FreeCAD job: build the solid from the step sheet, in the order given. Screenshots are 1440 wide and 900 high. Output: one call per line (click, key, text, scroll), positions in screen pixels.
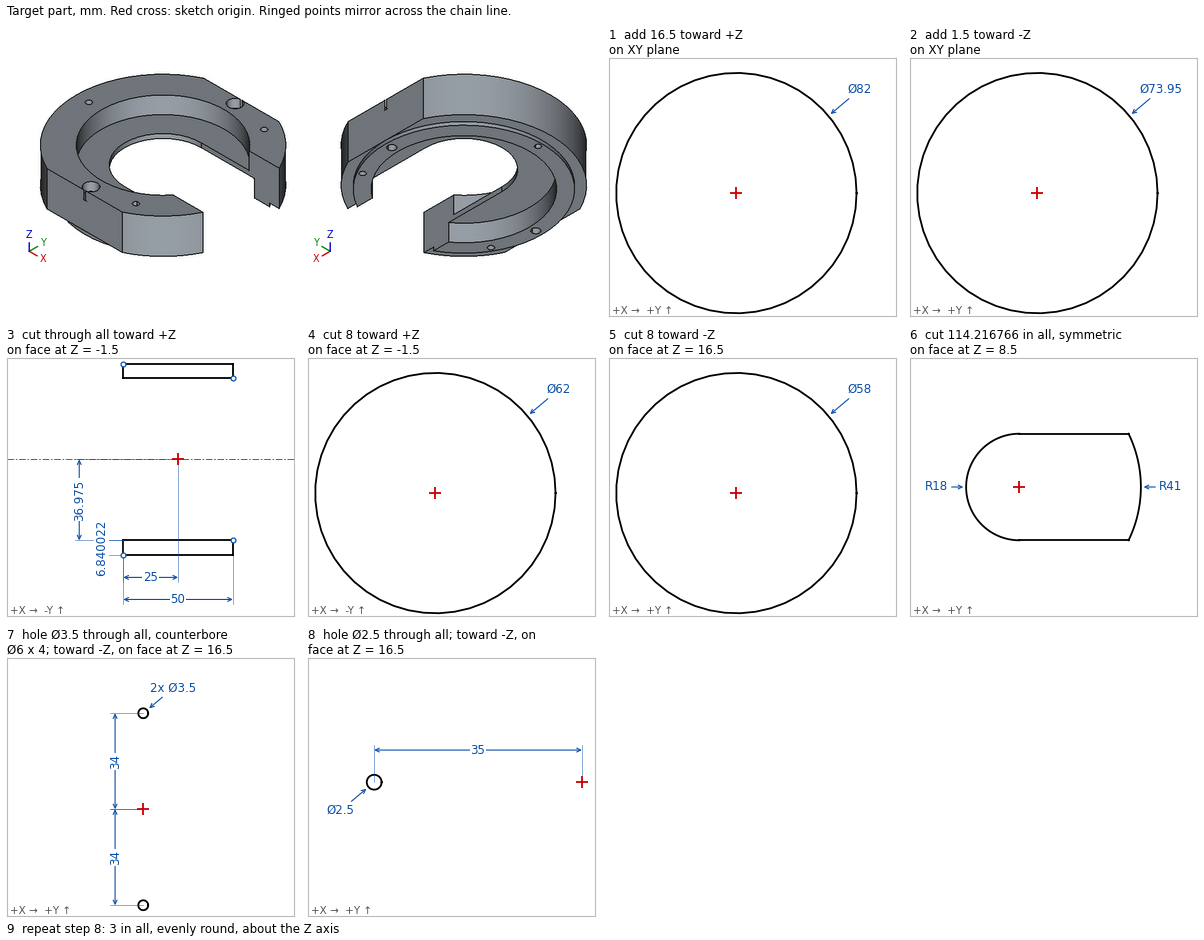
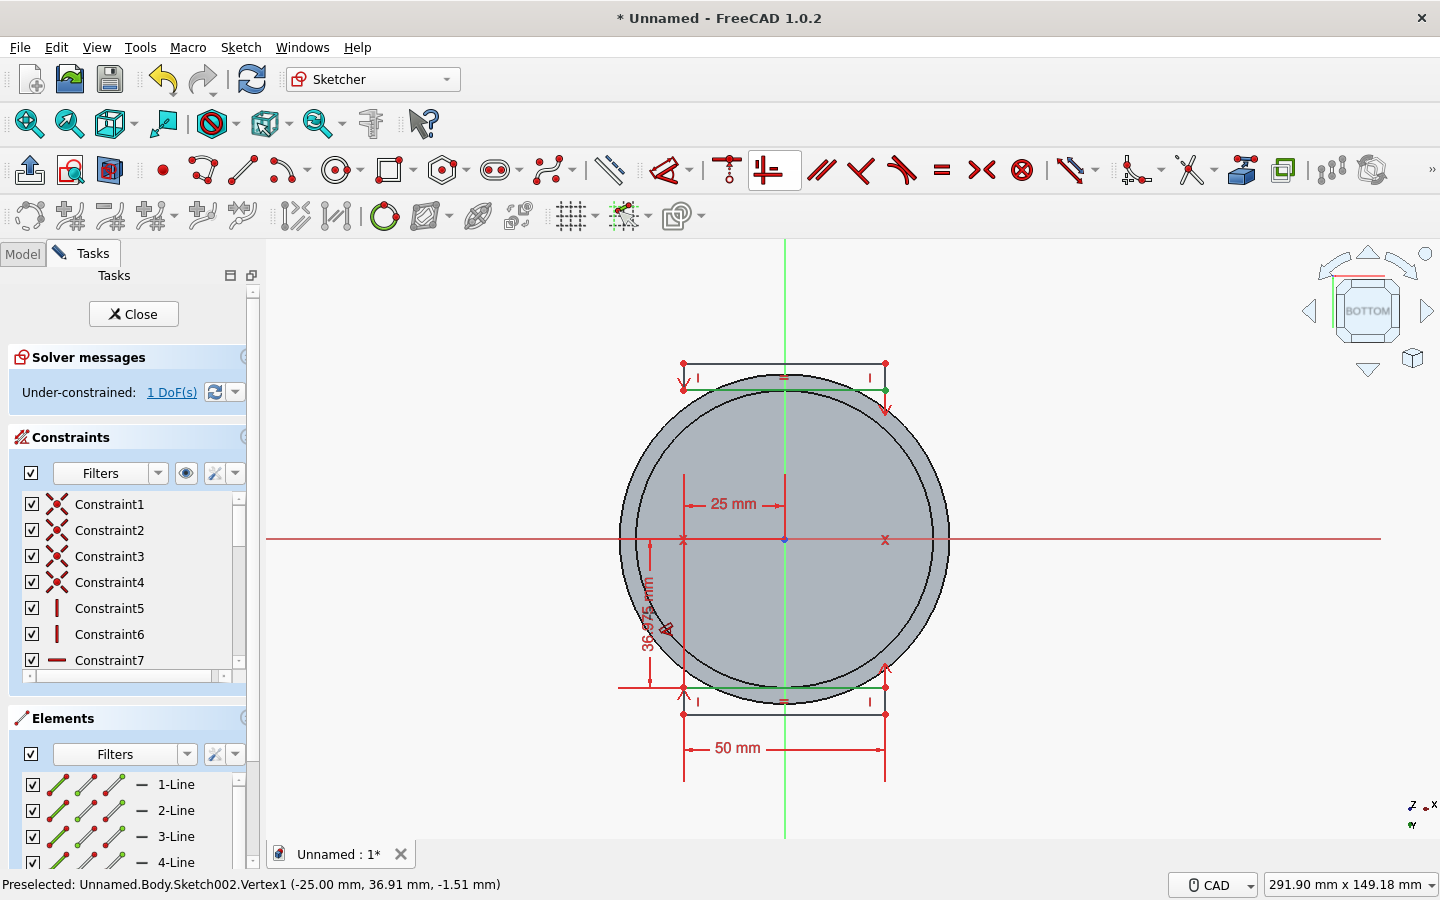
scroll(684, 699, up, 2)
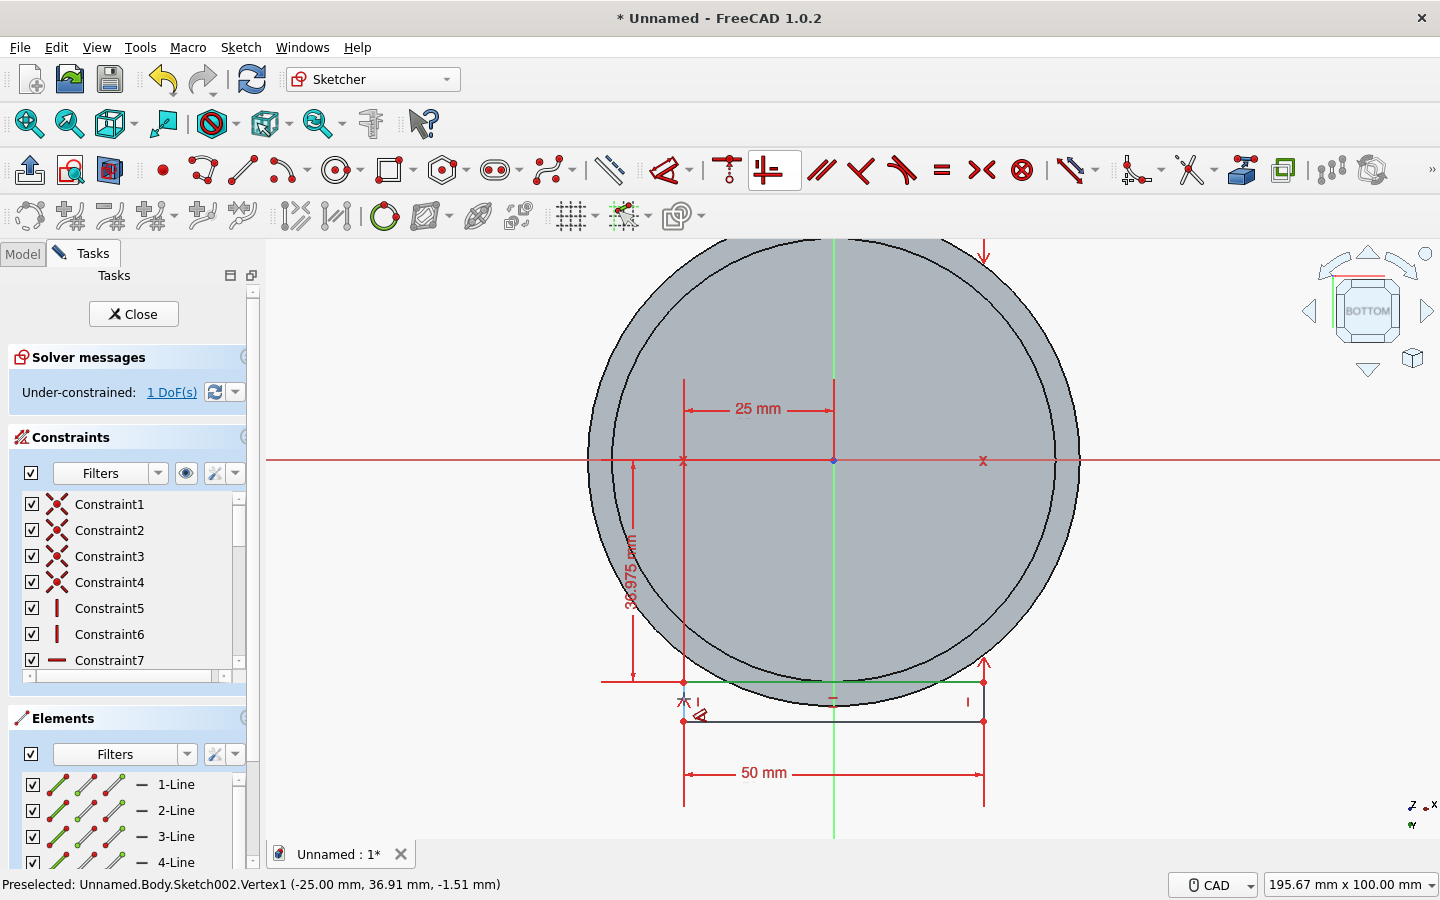
click(684, 698)
click(650, 702)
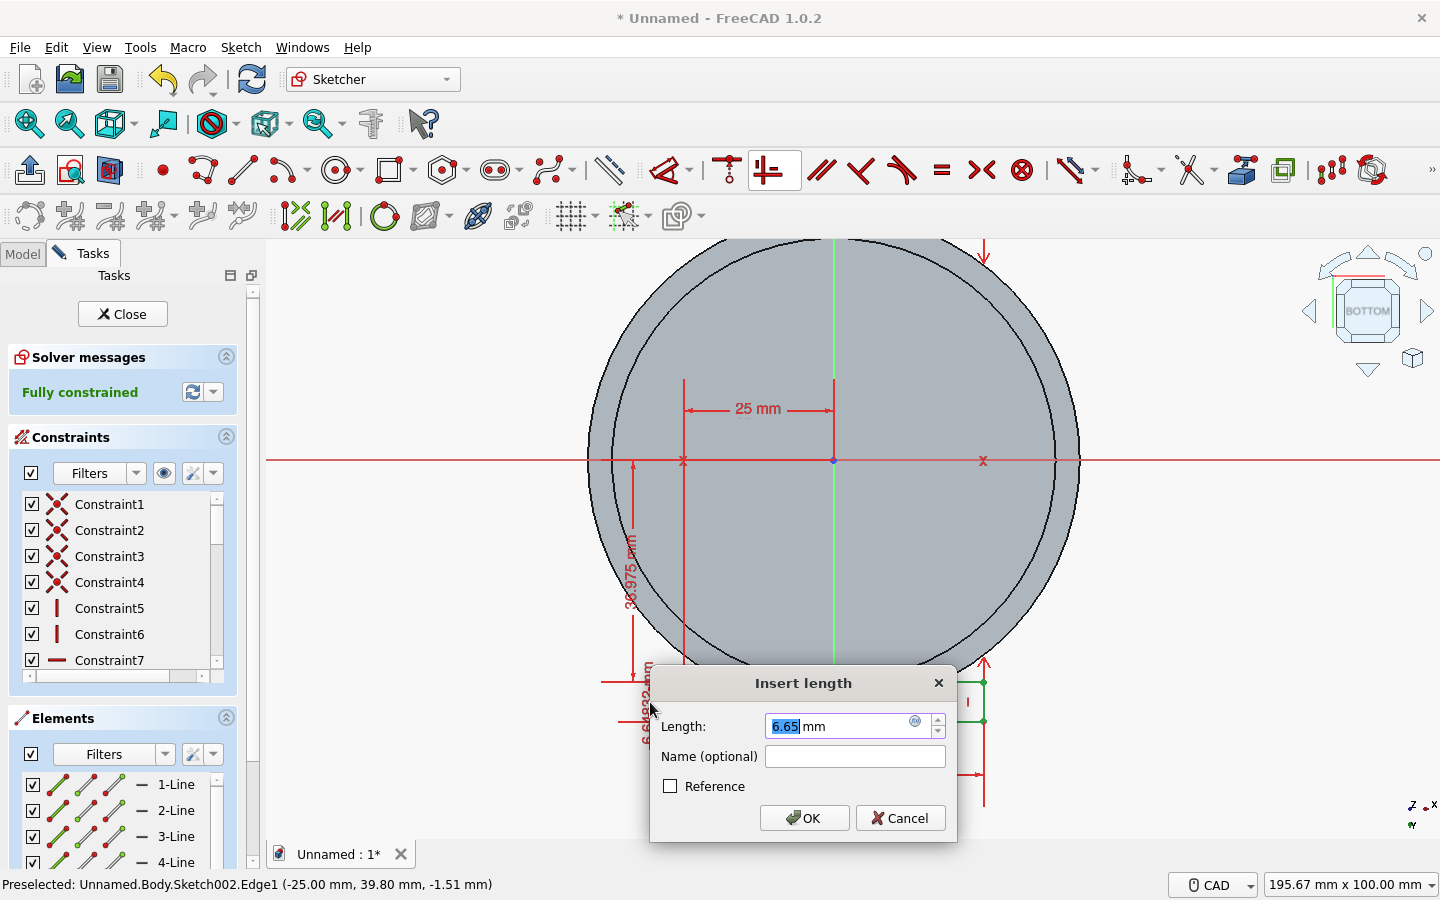
text(6.840022)
key(Return)
key(Escape)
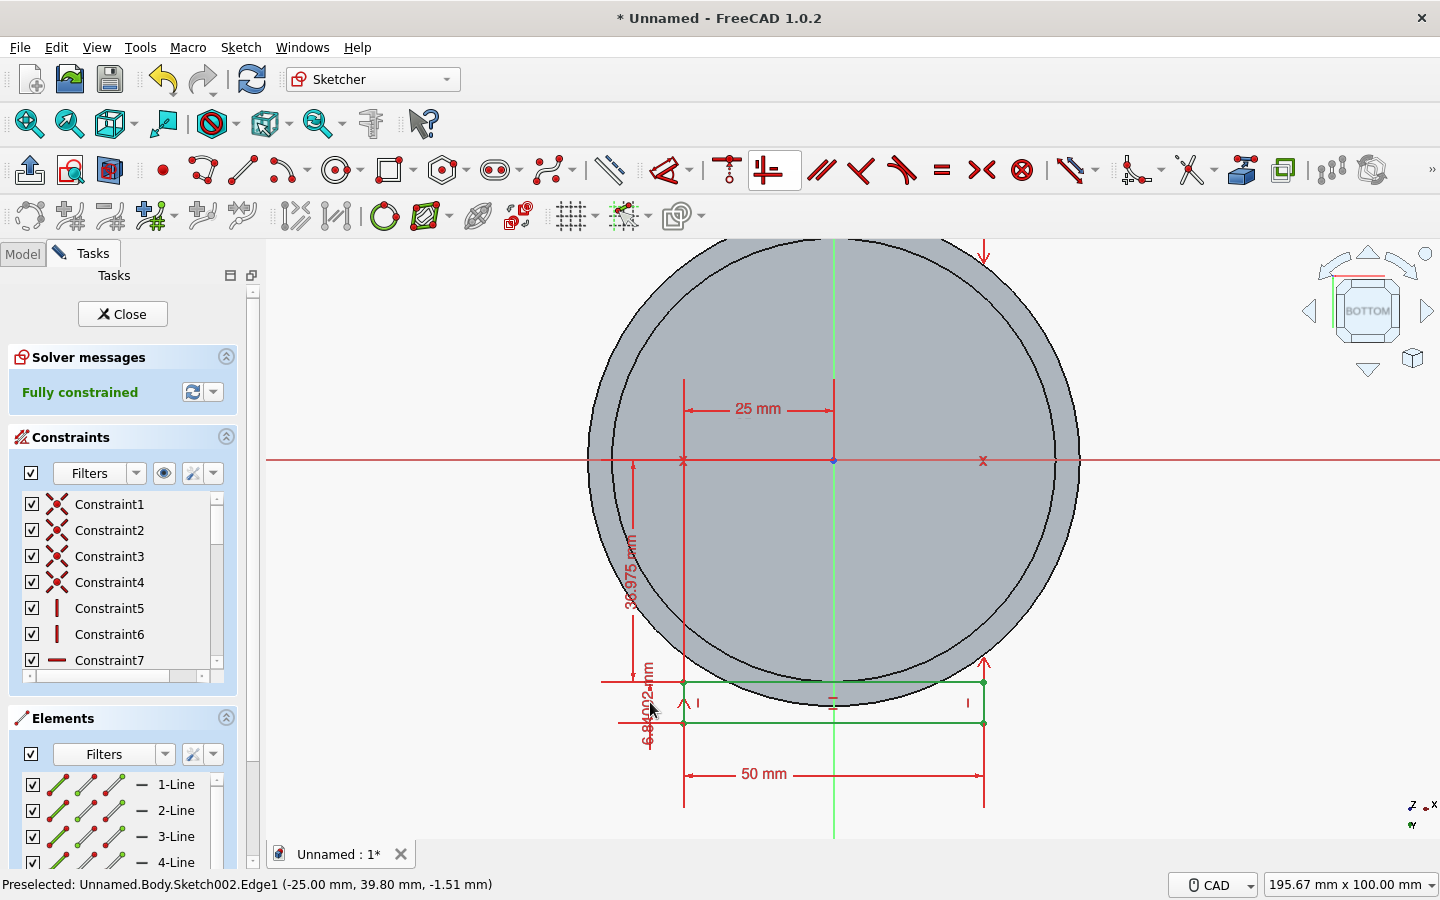
click(123, 314)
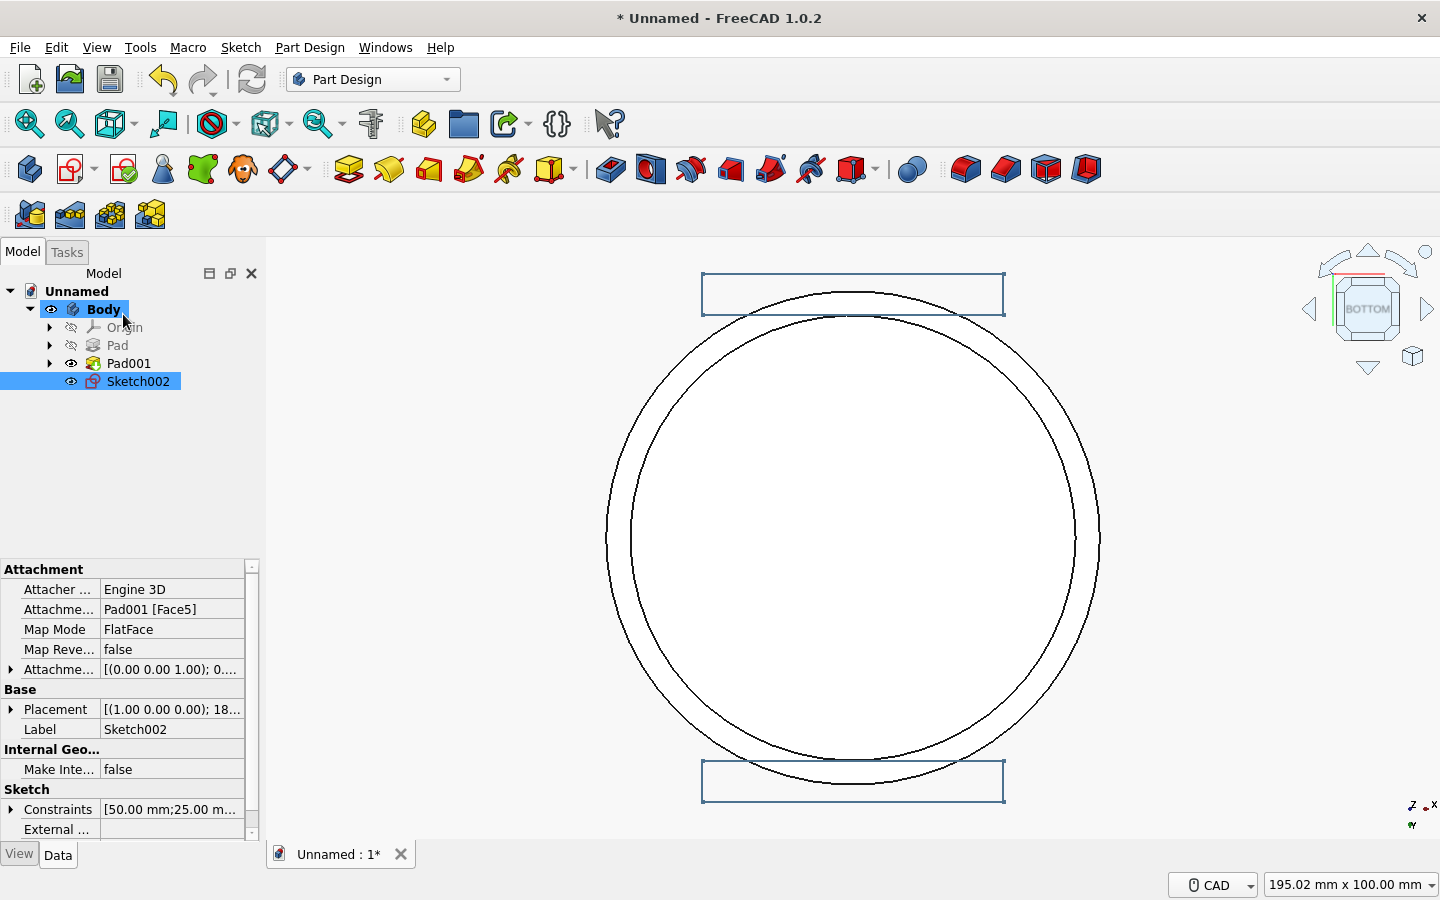
click(612, 170)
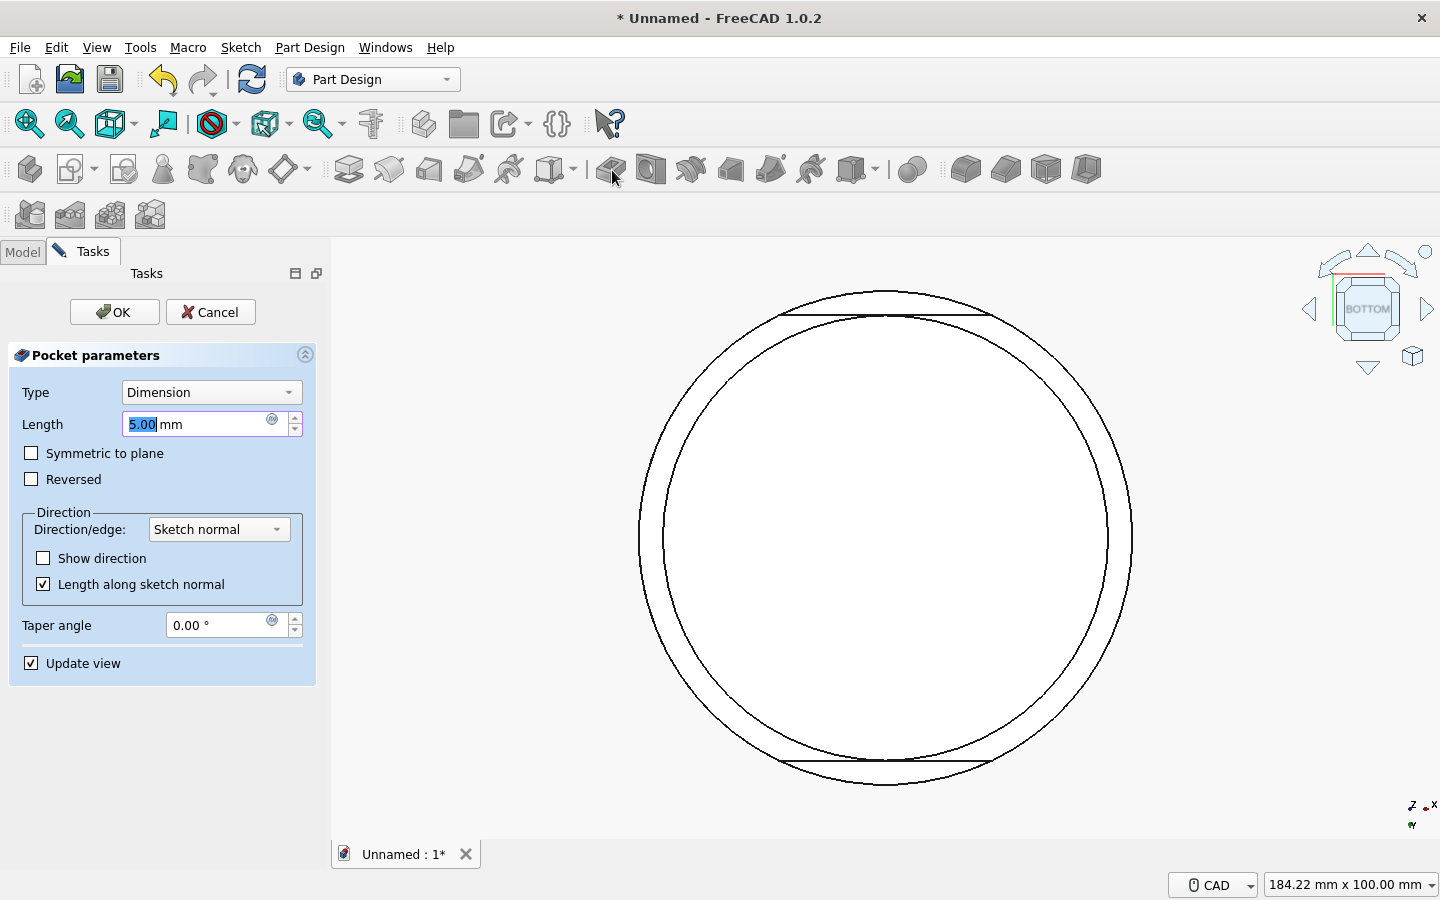
click(212, 392)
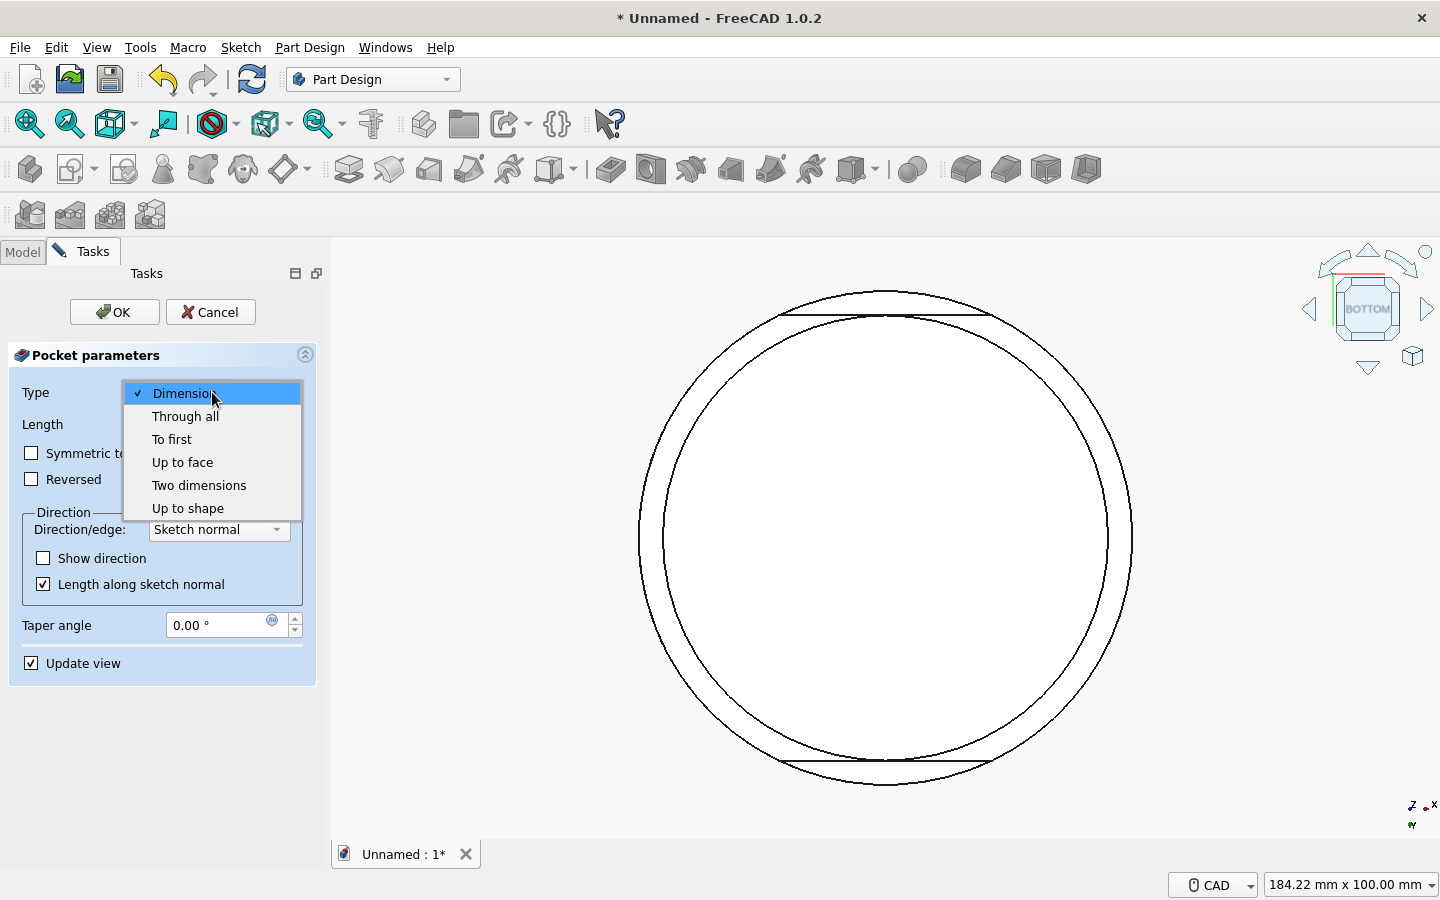
click(212, 416)